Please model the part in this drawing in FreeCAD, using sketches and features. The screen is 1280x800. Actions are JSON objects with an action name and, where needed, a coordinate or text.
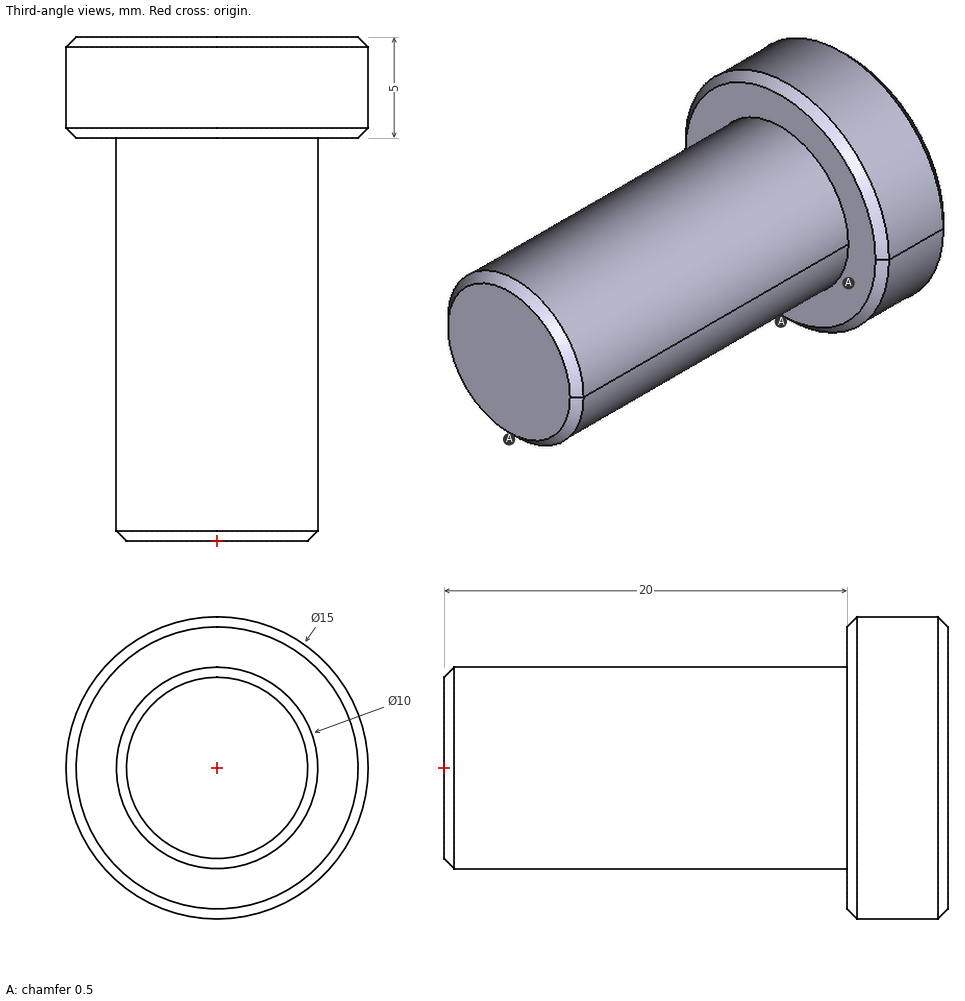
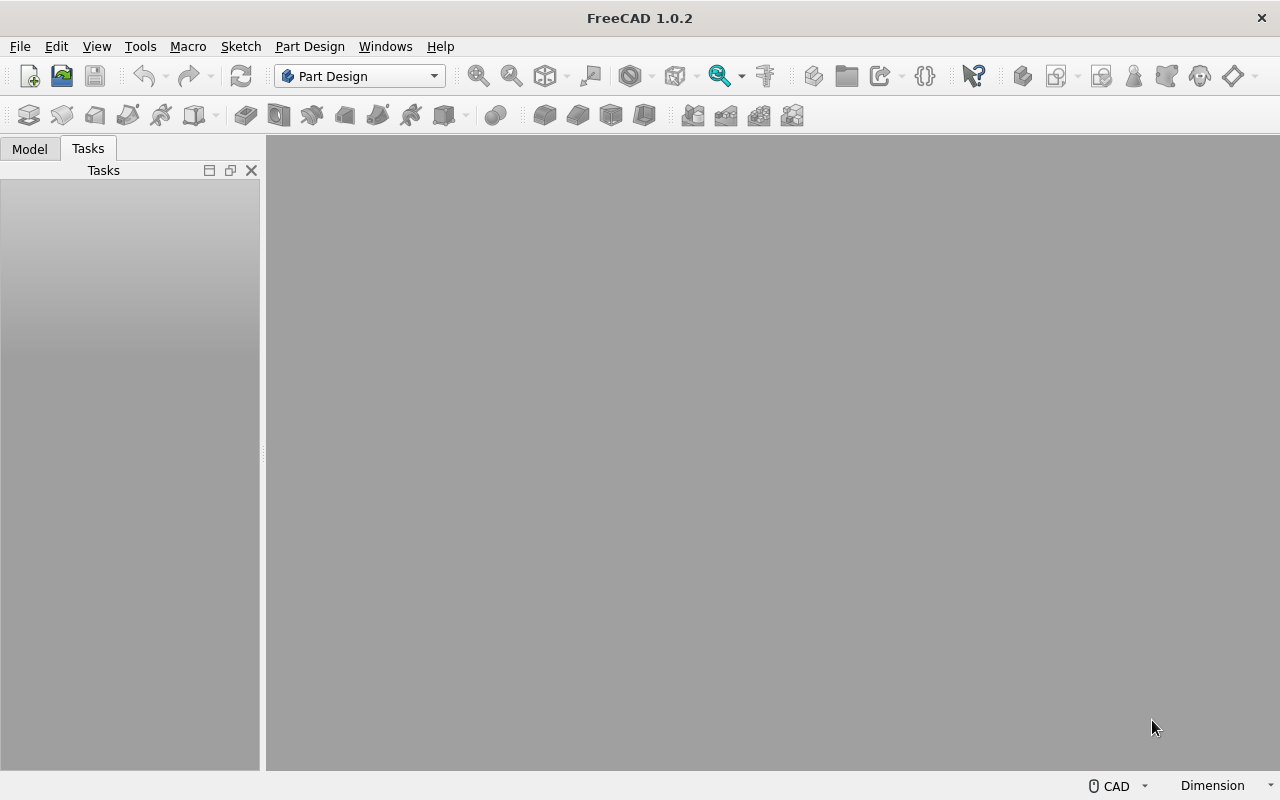
{"action": "key", "text": "ctrl+n"}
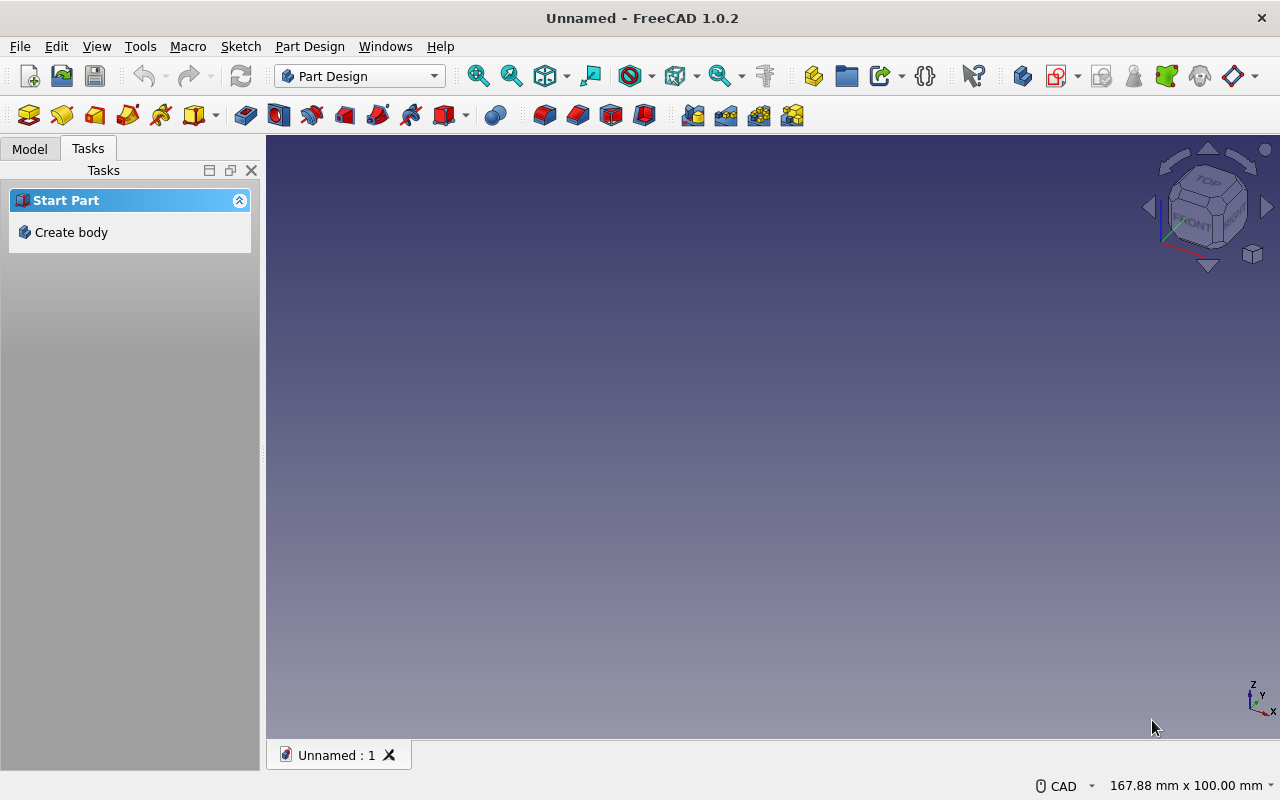
{"action": "left_click", "coordinate": [1056, 76]}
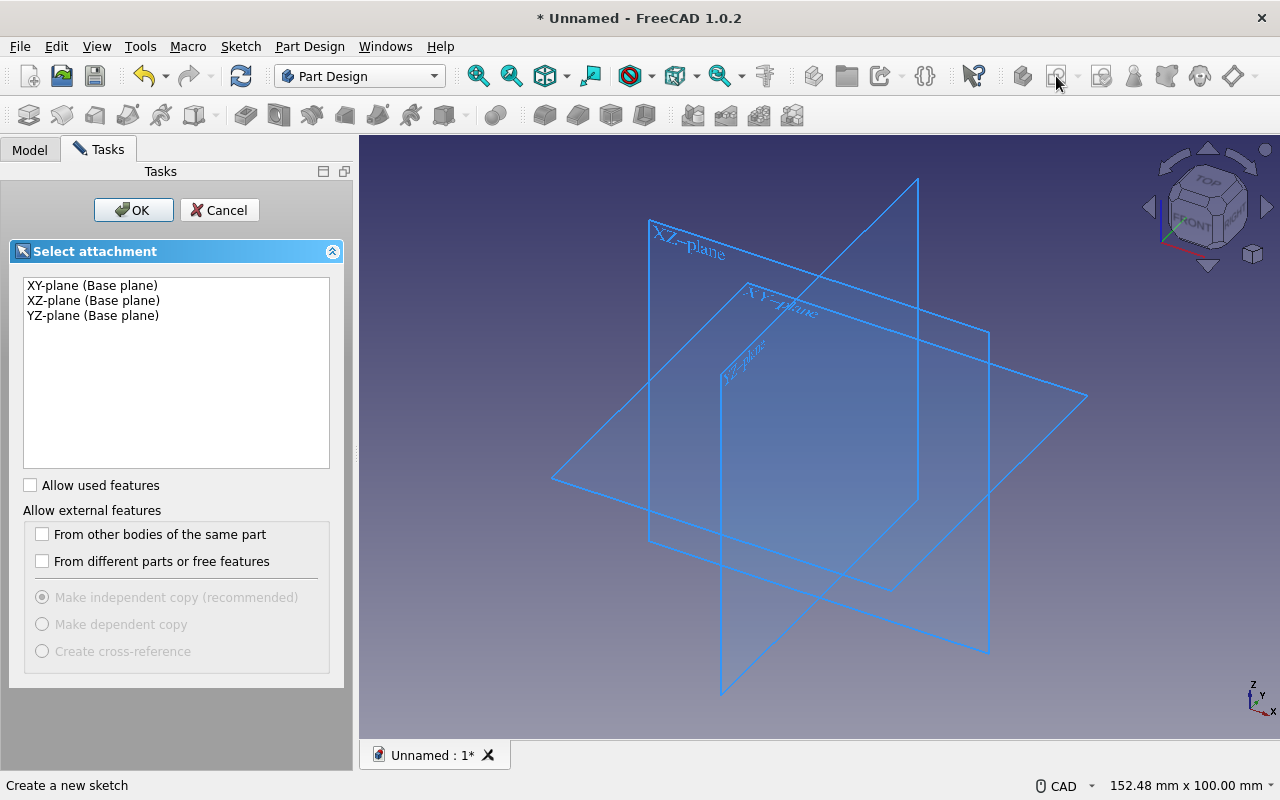
{"action": "left_click", "coordinate": [84, 300]}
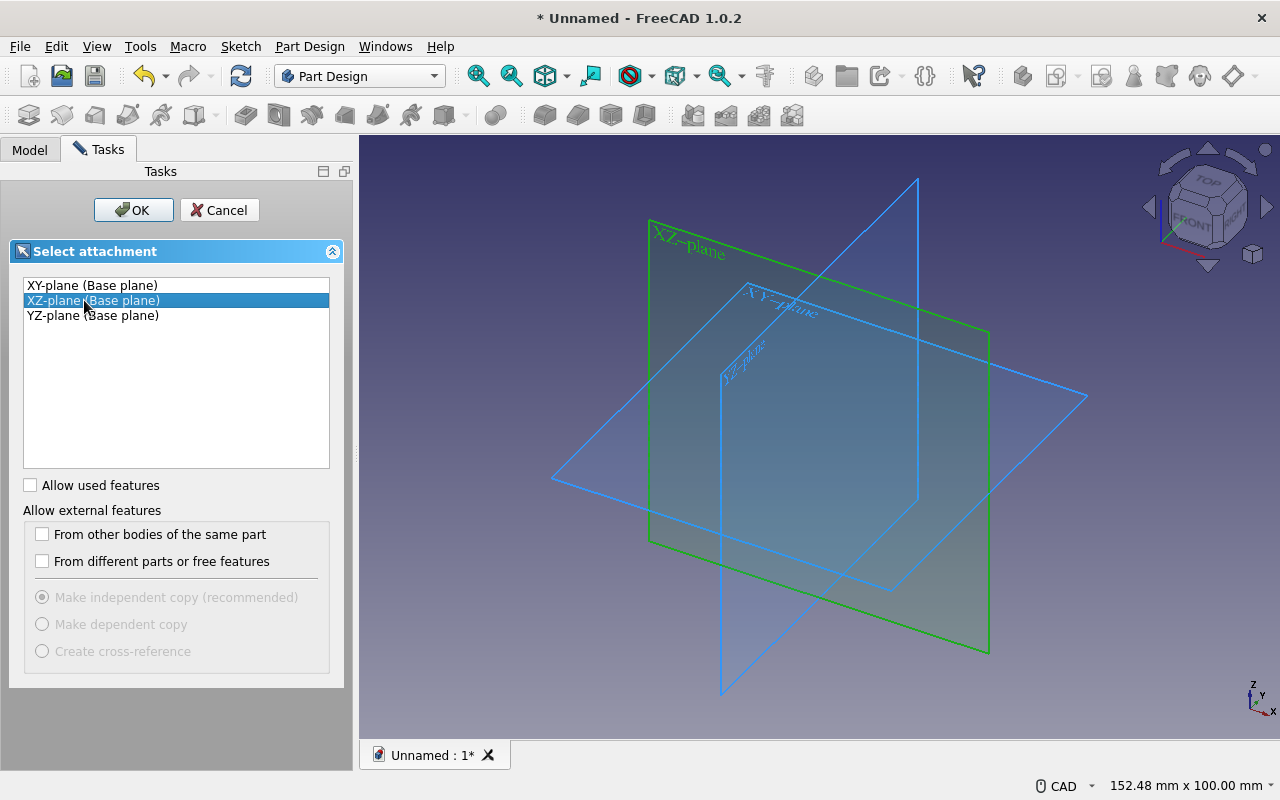
{"action": "left_click", "coordinate": [134, 210]}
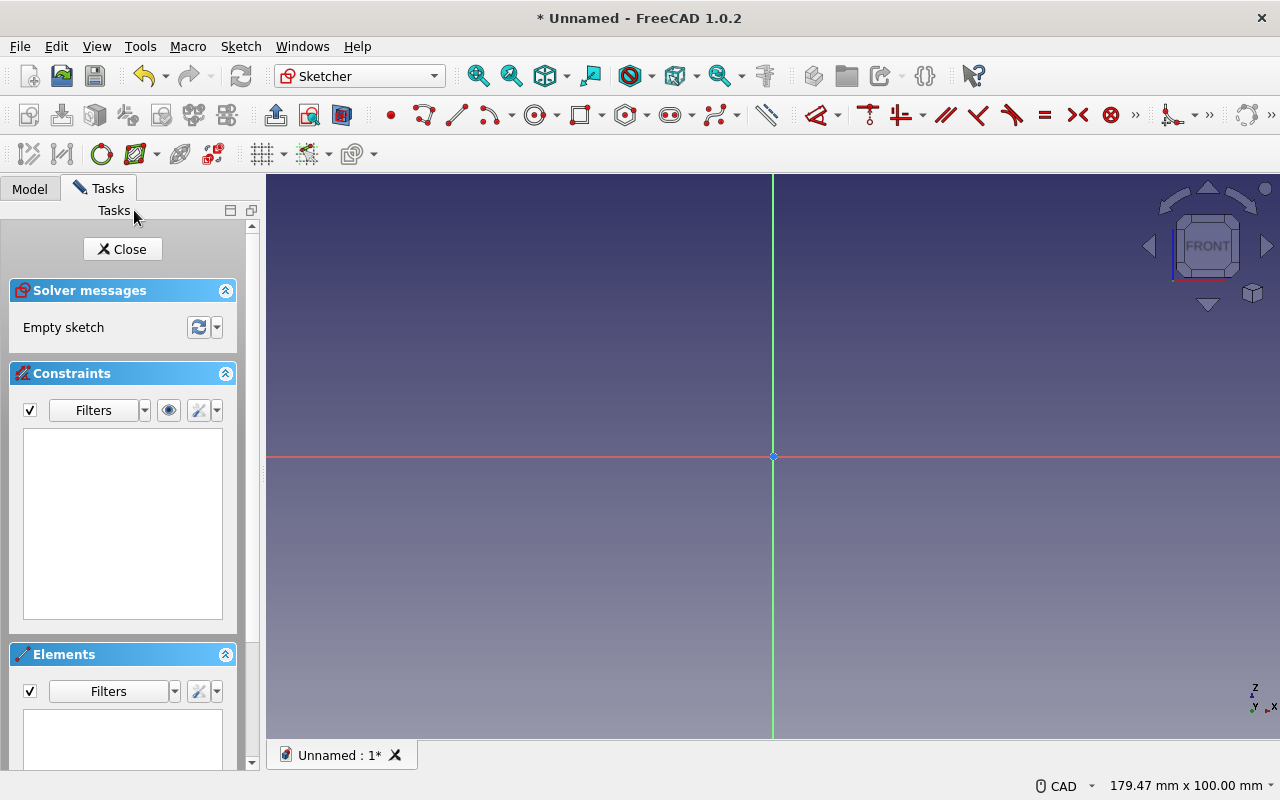
{"action": "scroll", "coordinate": [787, 456], "scroll_direction": "up", "scroll_amount": 9}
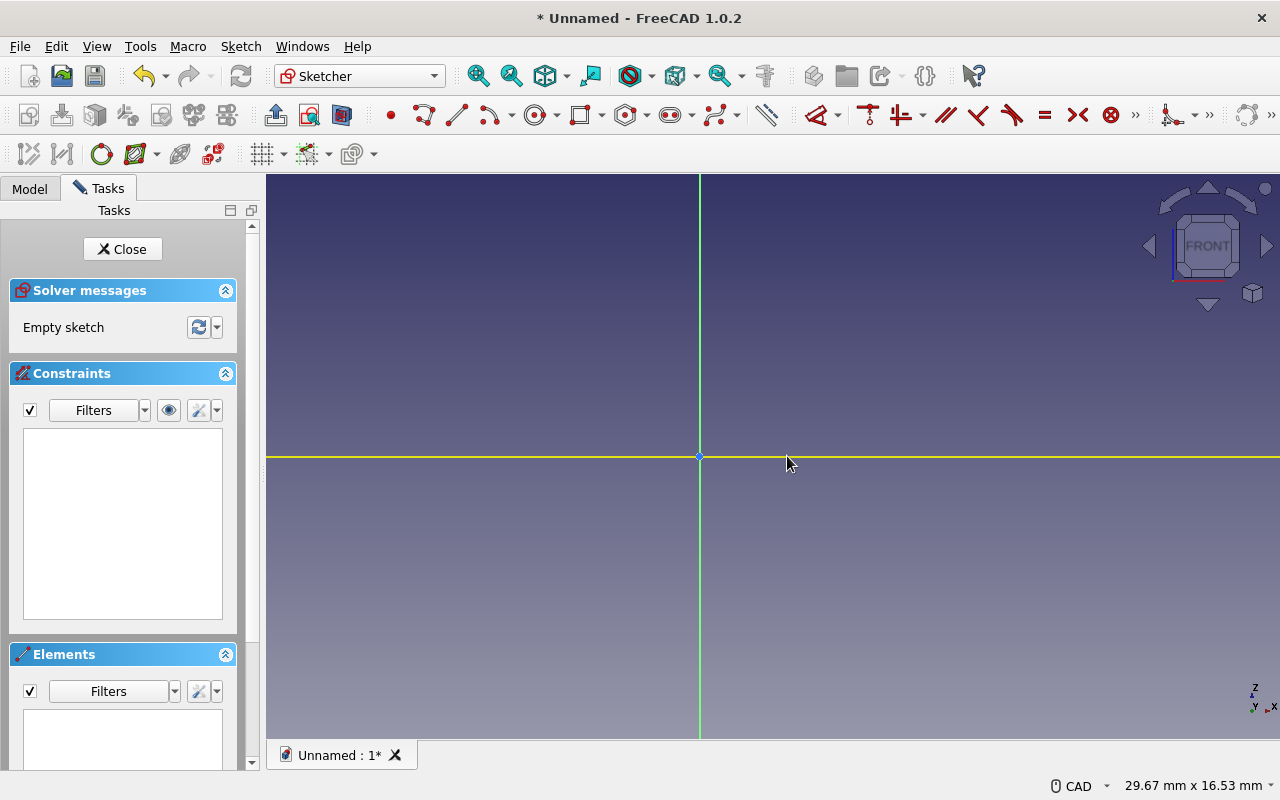
{"action": "left_click", "coordinate": [534, 116]}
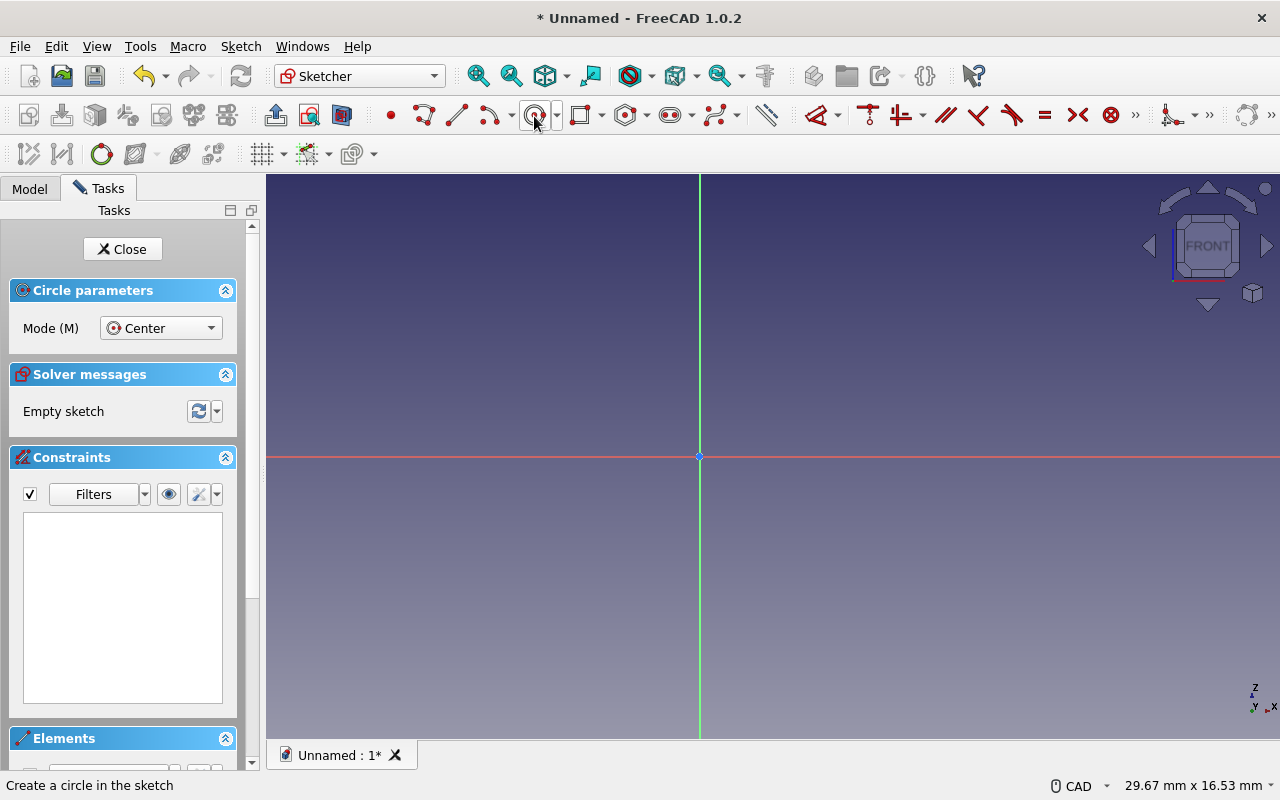
{"action": "left_click", "coordinate": [700, 456]}
{"action": "mouse_move", "coordinate": [821, 336]}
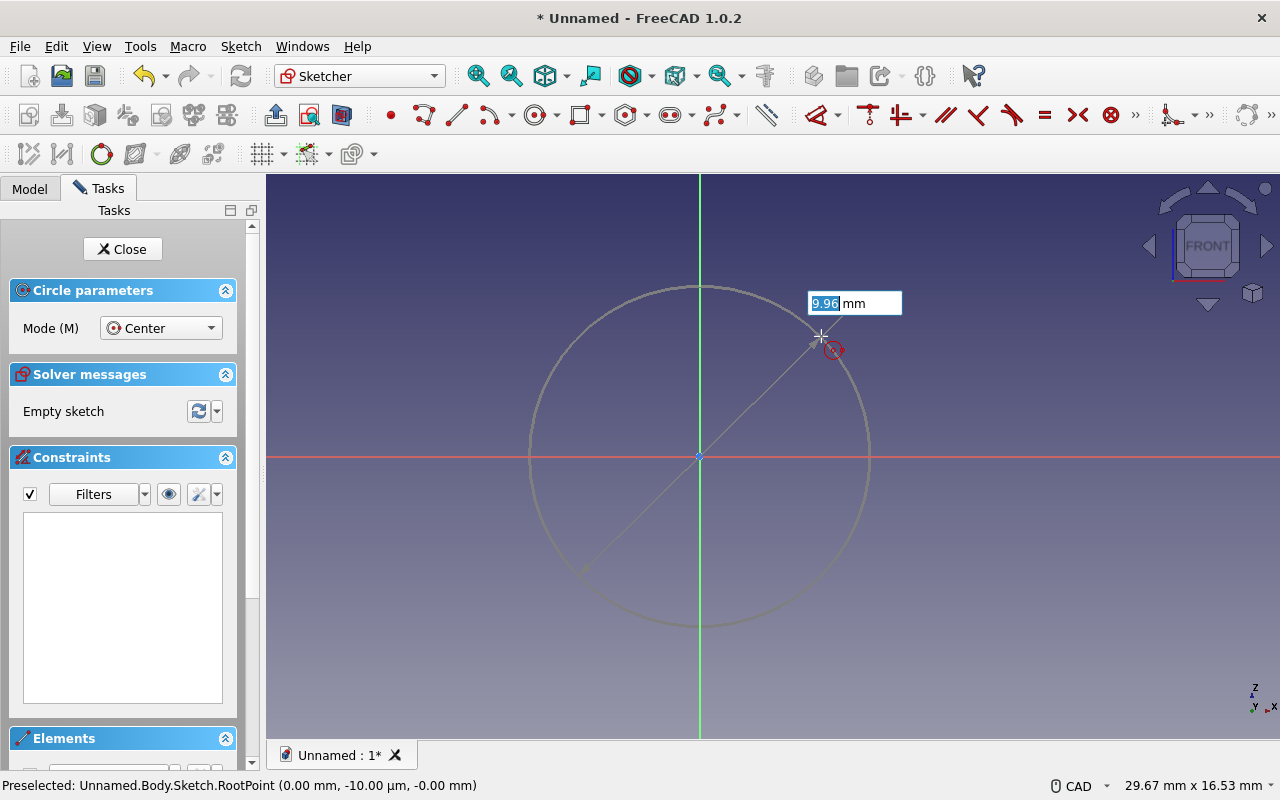
{"action": "type", "text": "10"}
{"action": "key", "text": "Return"}
{"action": "key", "text": "Escape"}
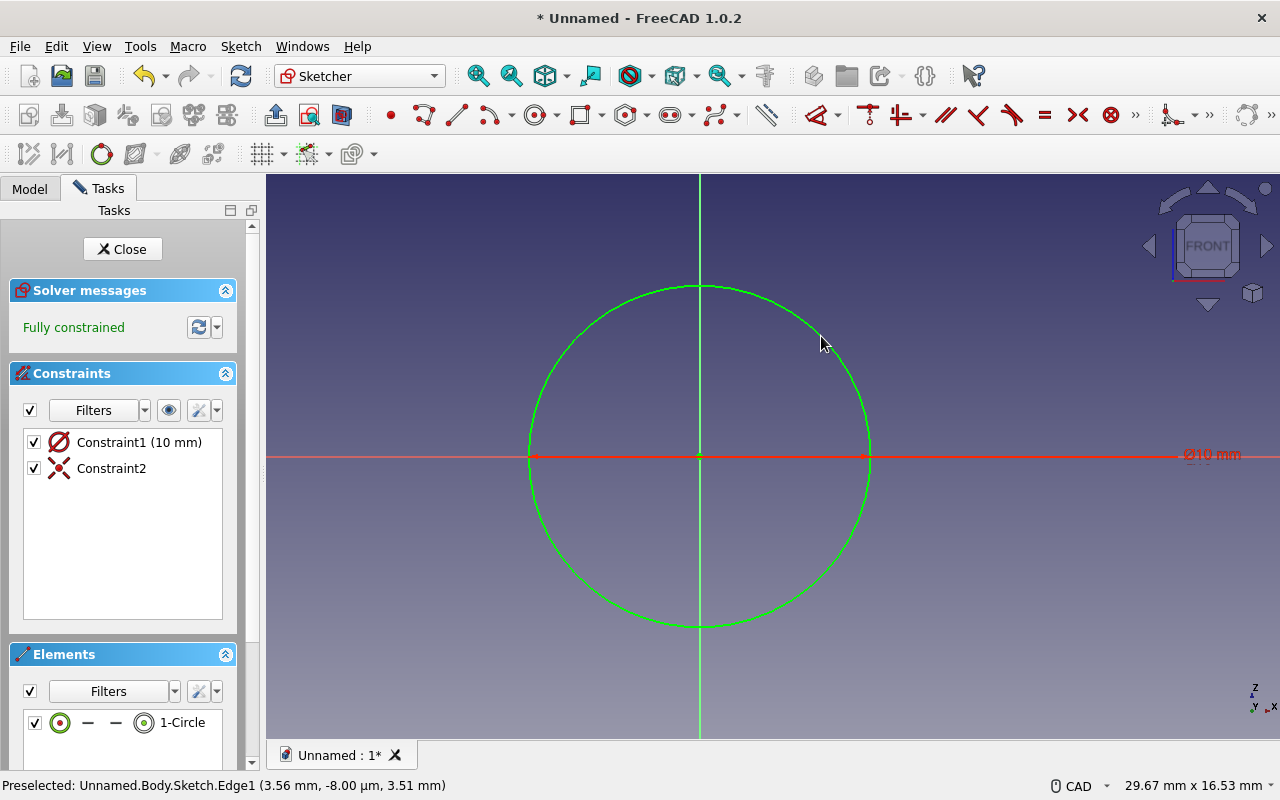
{"action": "left_click", "coordinate": [123, 249]}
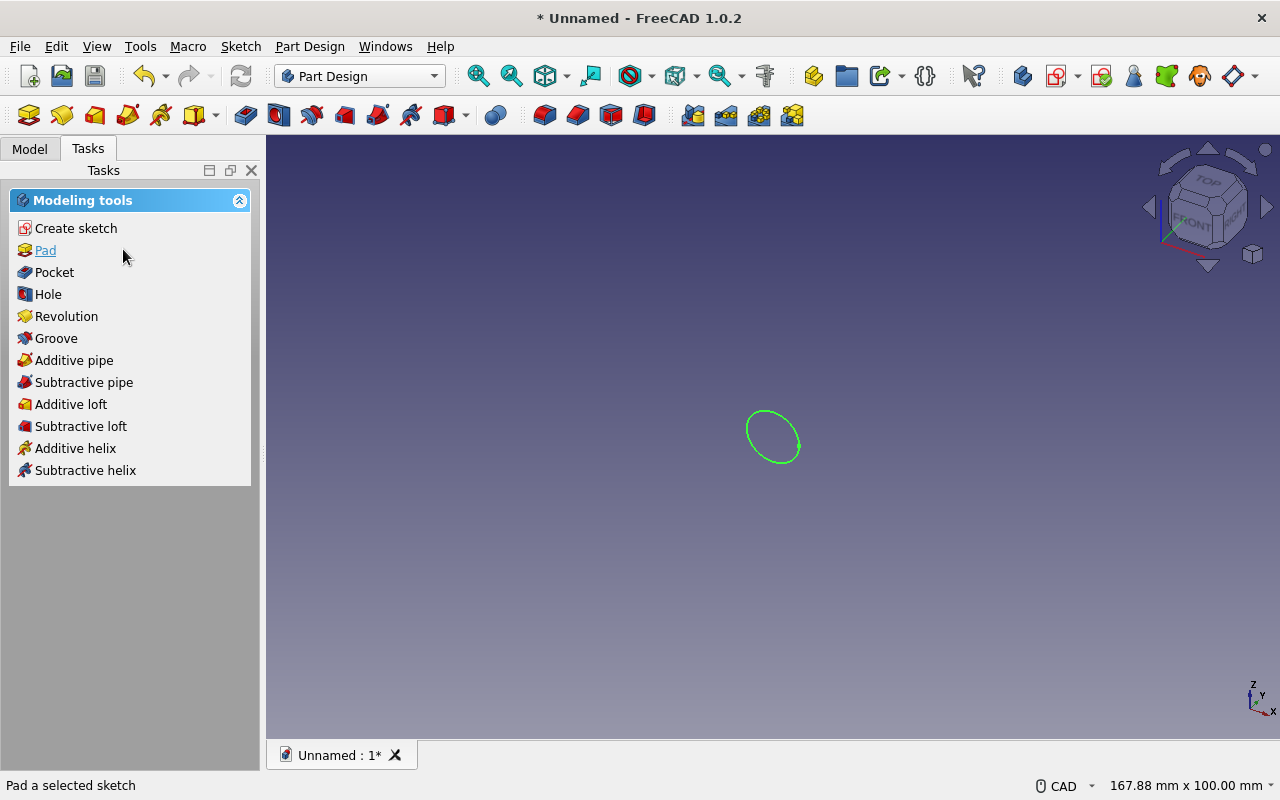
{"action": "left_click", "coordinate": [29, 116]}